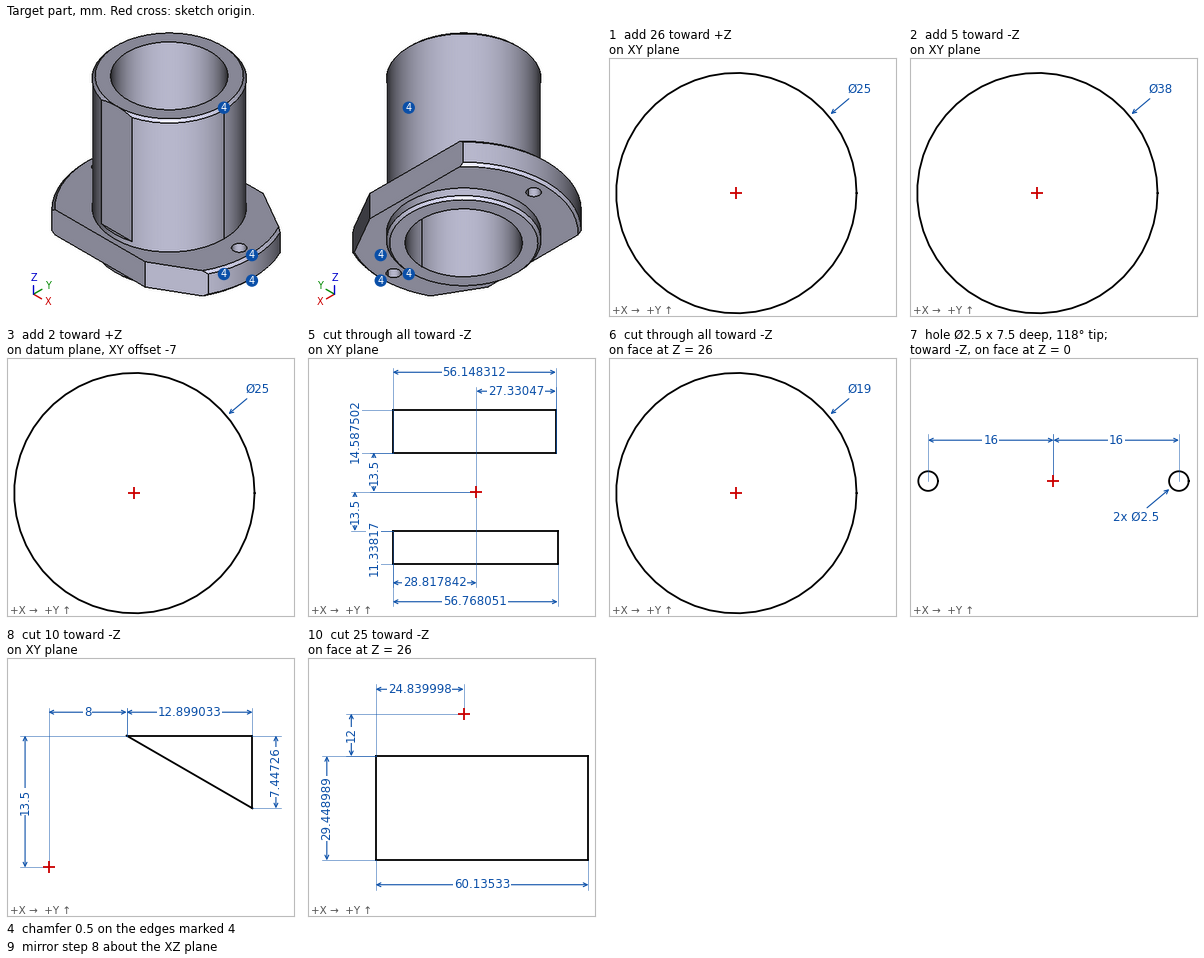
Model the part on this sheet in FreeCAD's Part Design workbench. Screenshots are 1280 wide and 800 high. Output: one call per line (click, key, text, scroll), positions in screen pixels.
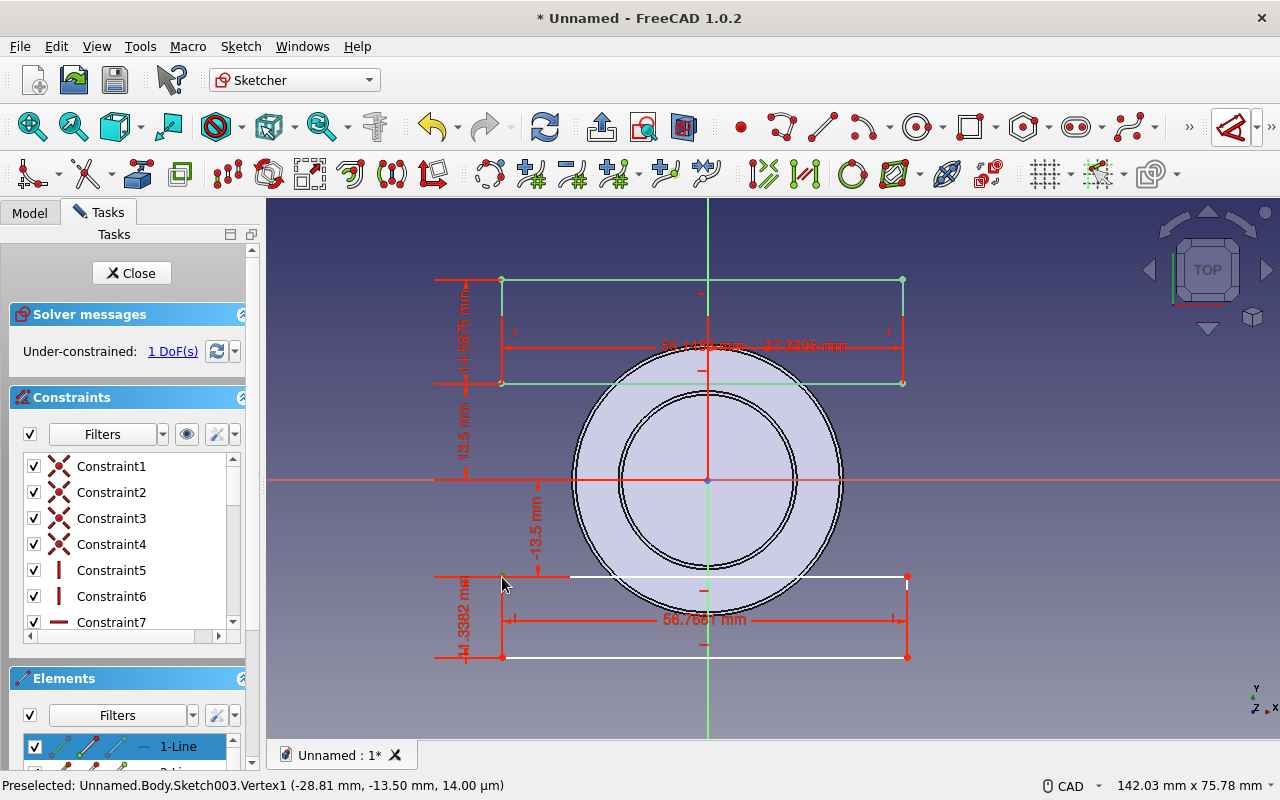
key(l)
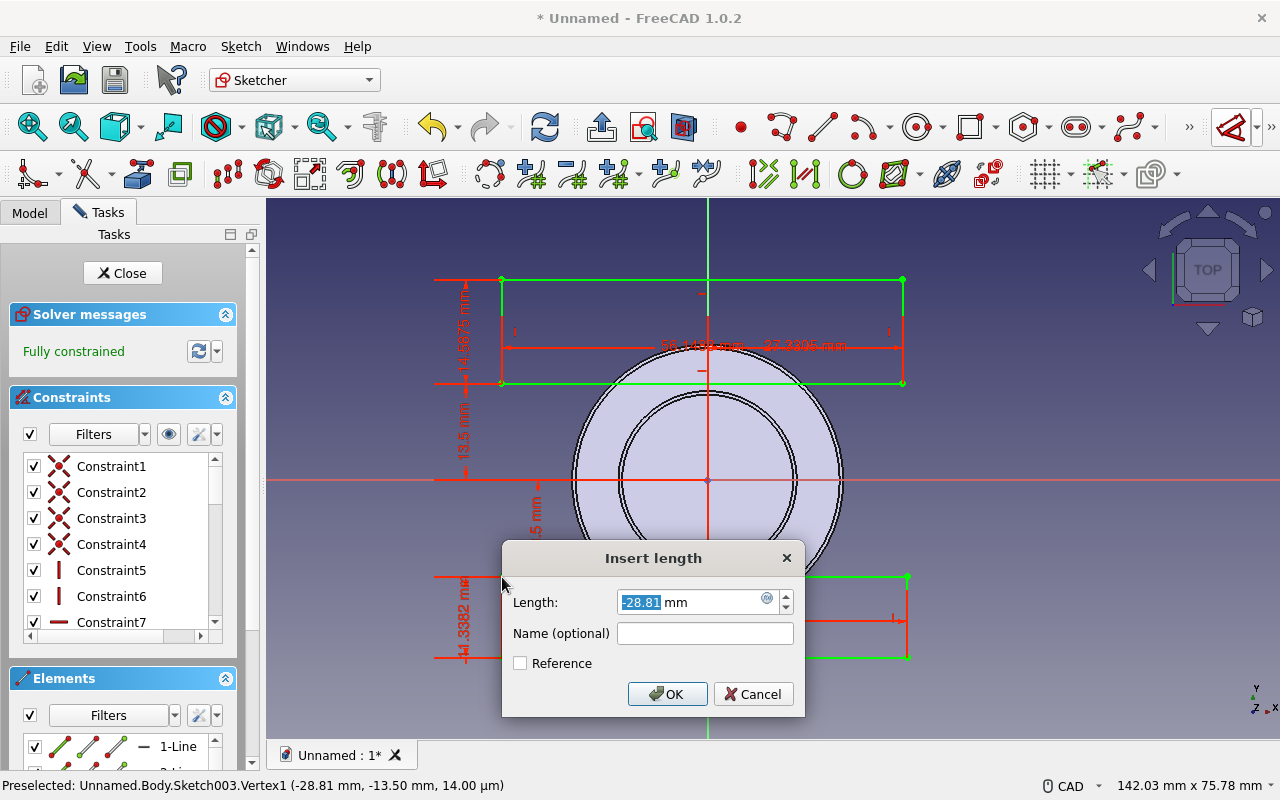
text(-28.817842)
key(Return)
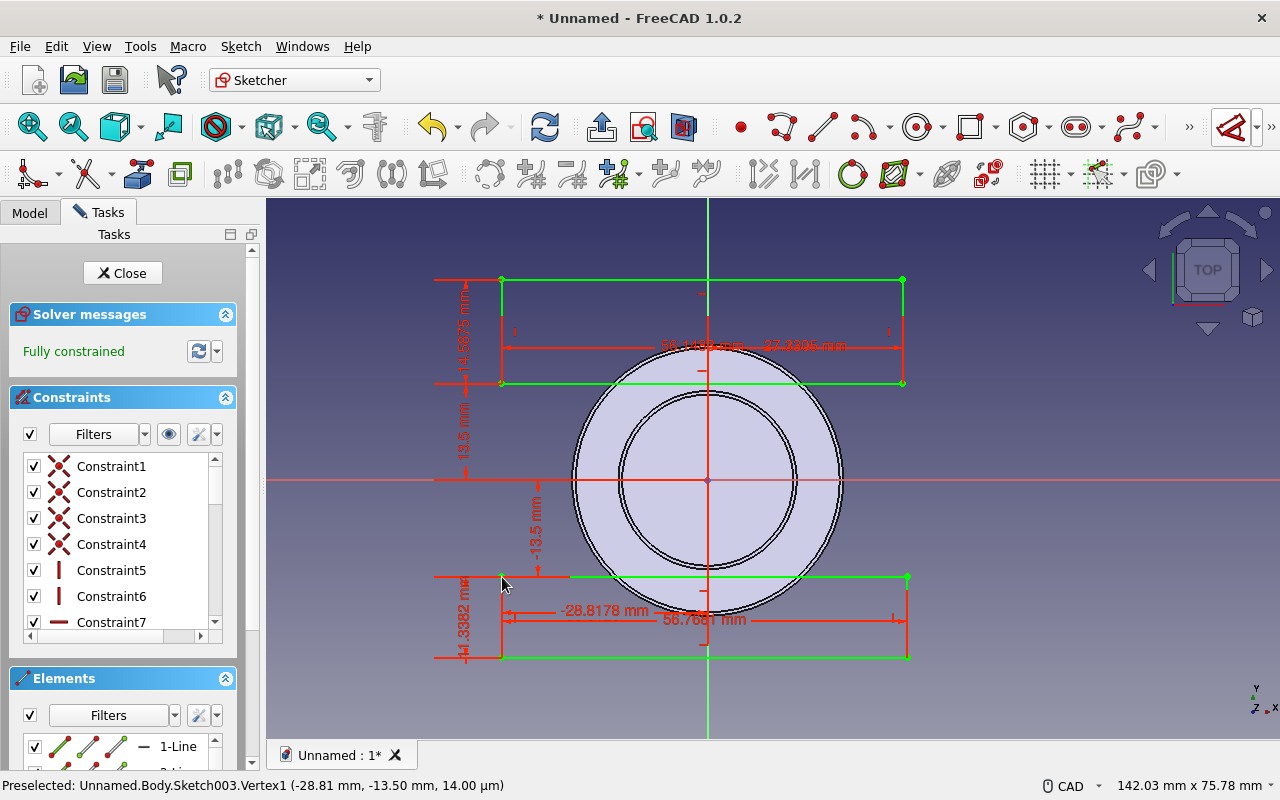
click(123, 273)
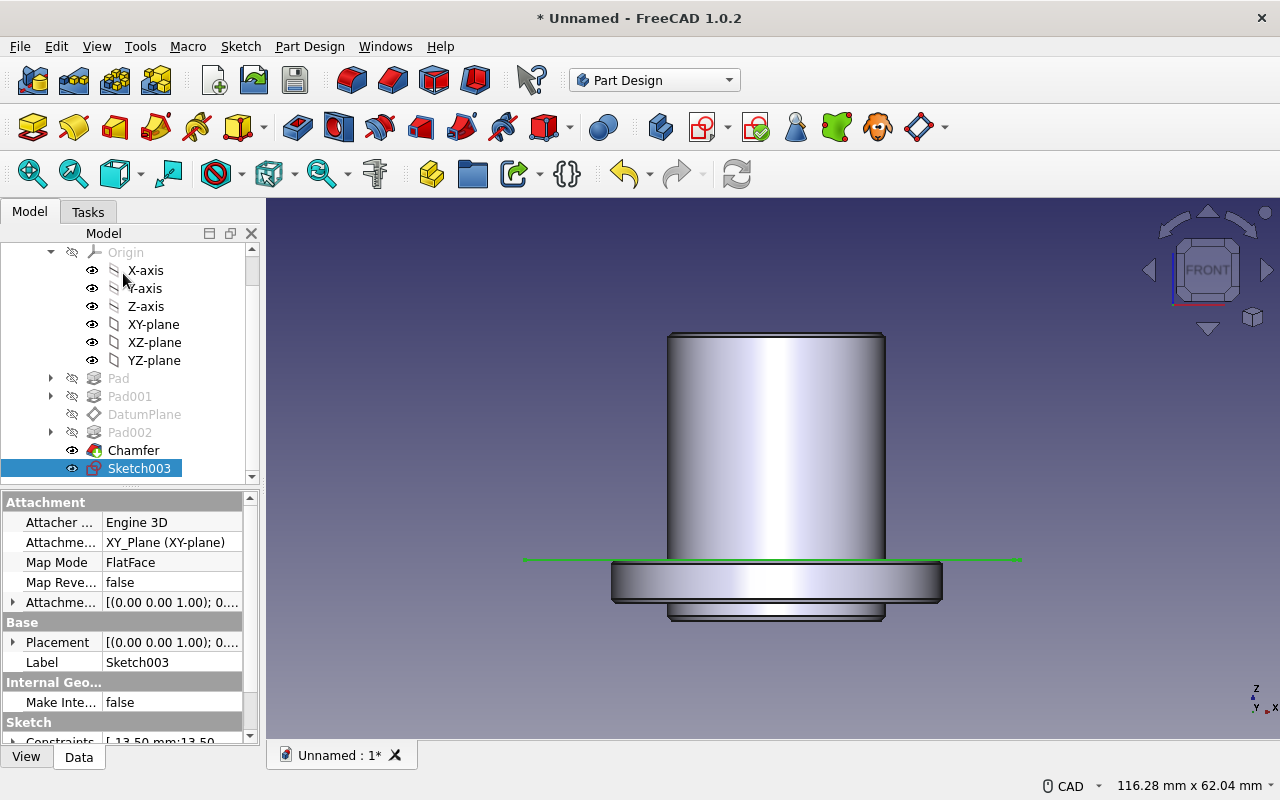
click(298, 128)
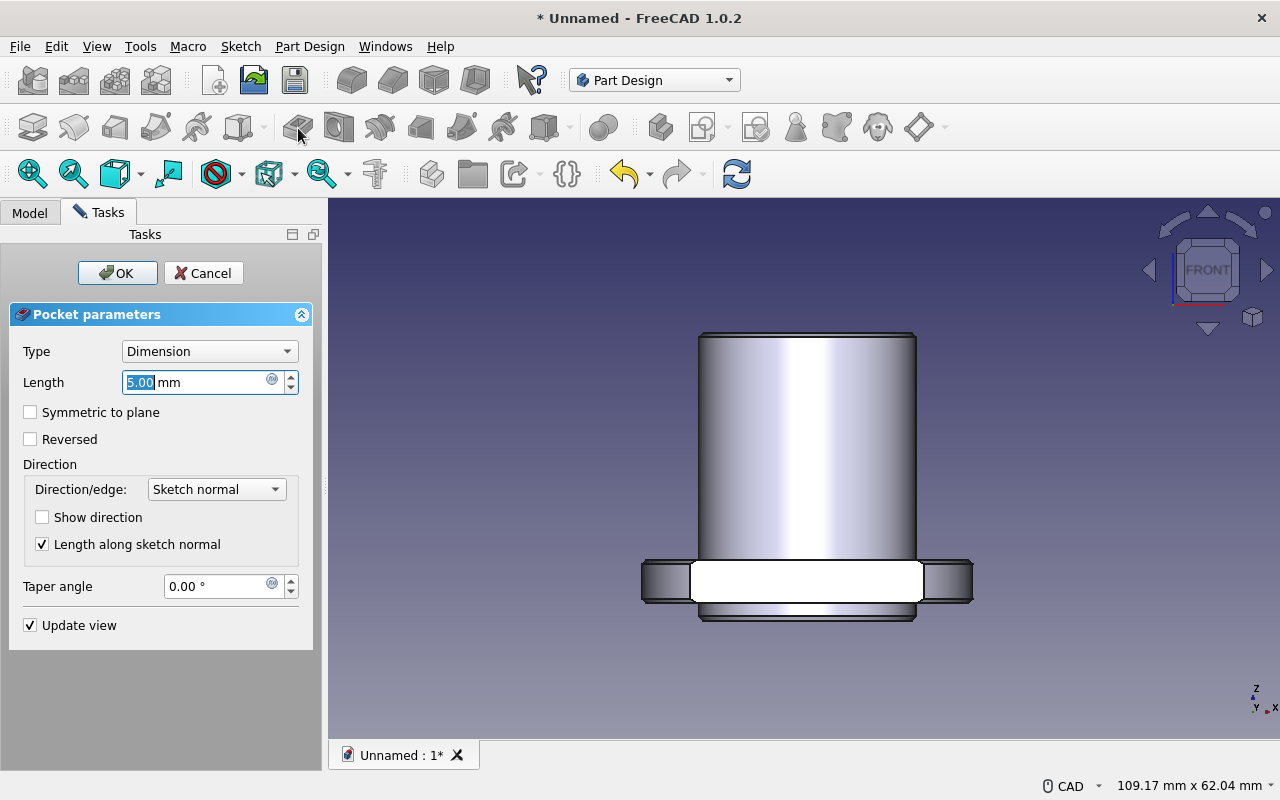
click(210, 352)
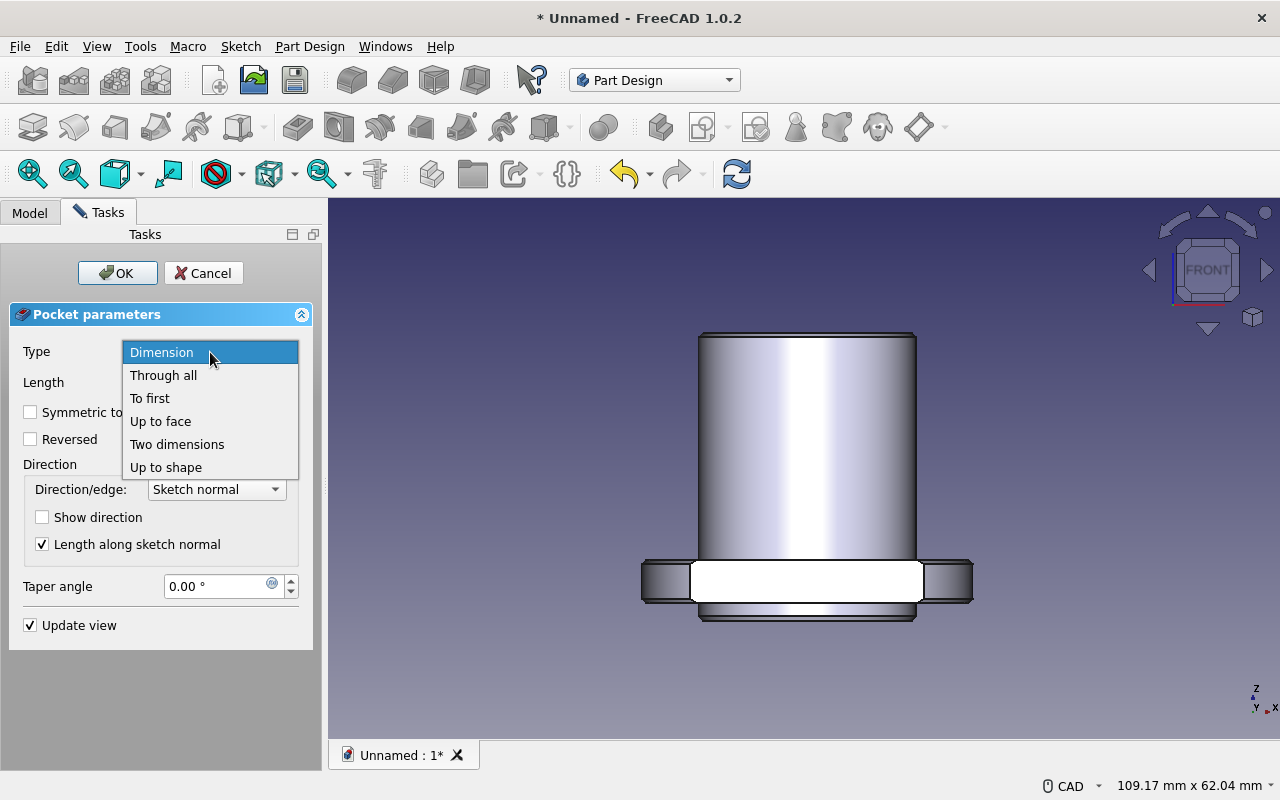
click(208, 376)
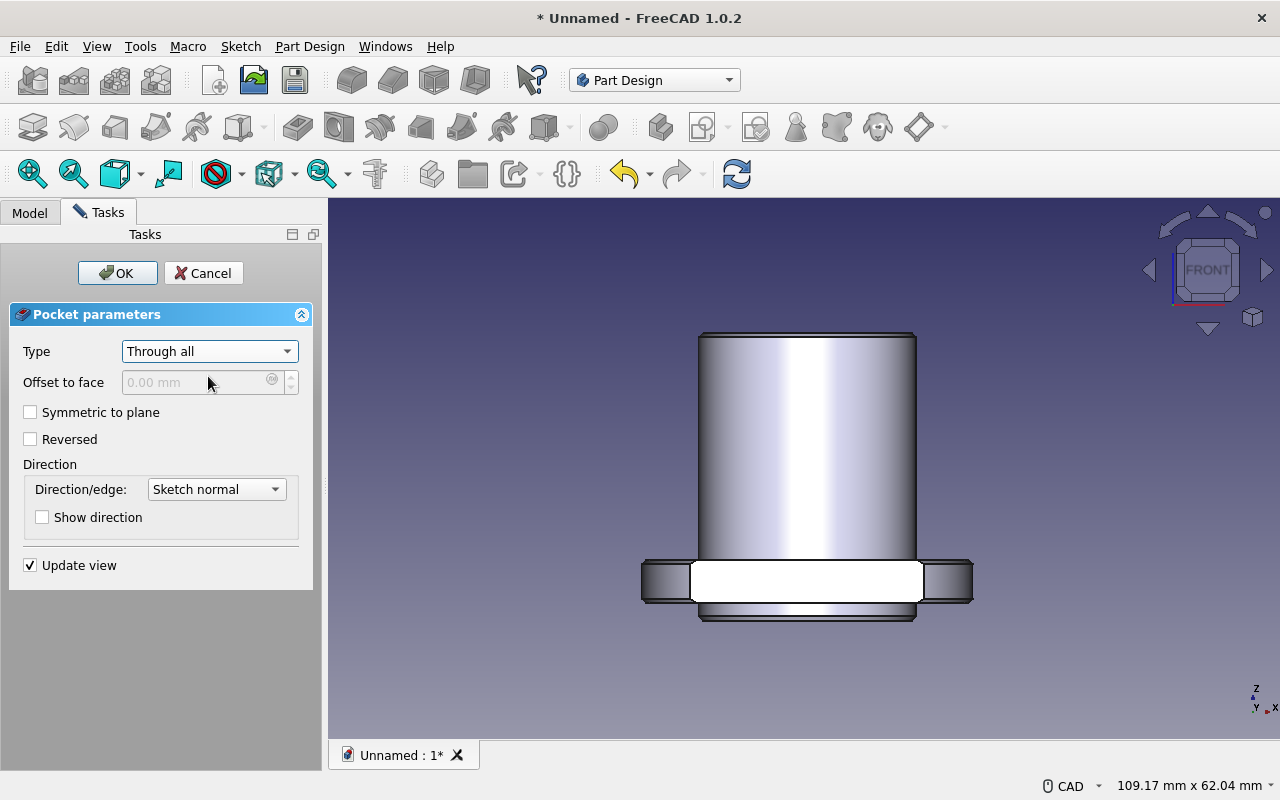
click(118, 273)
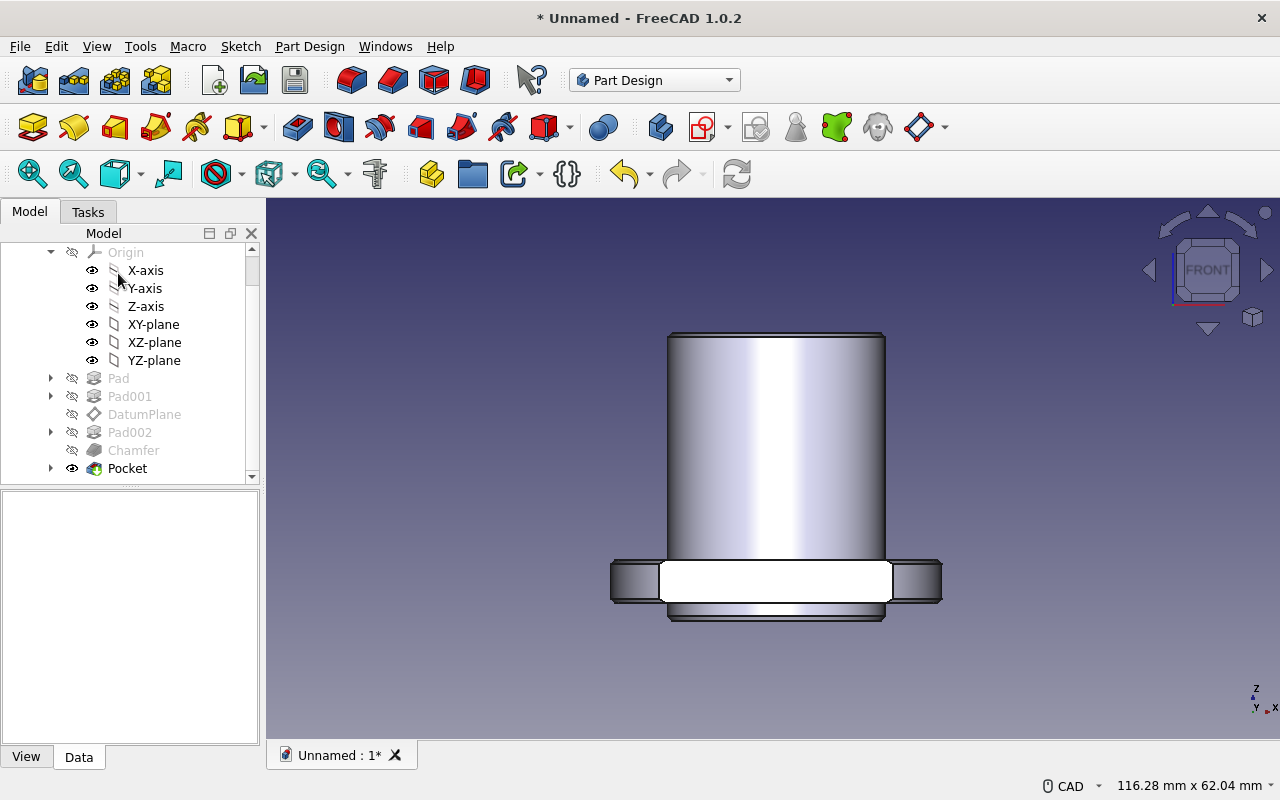
key(0)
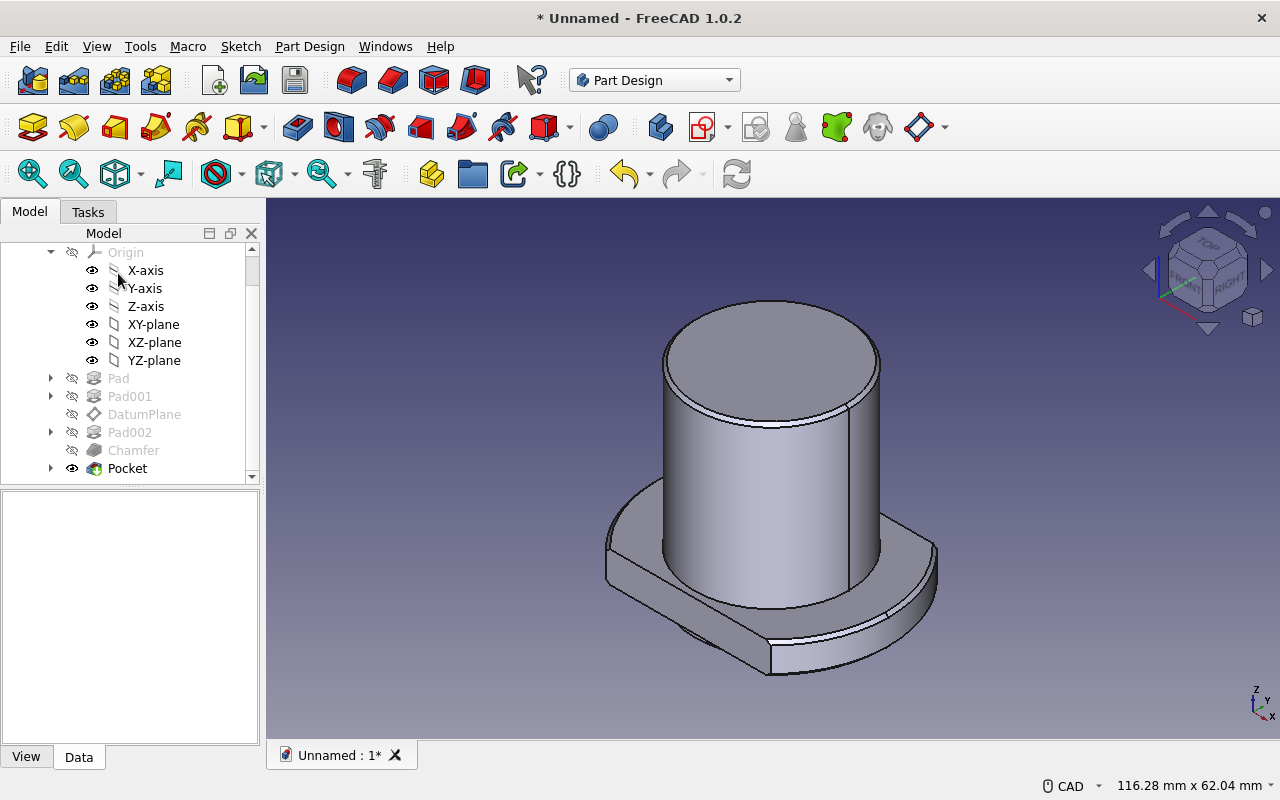
click(771, 360)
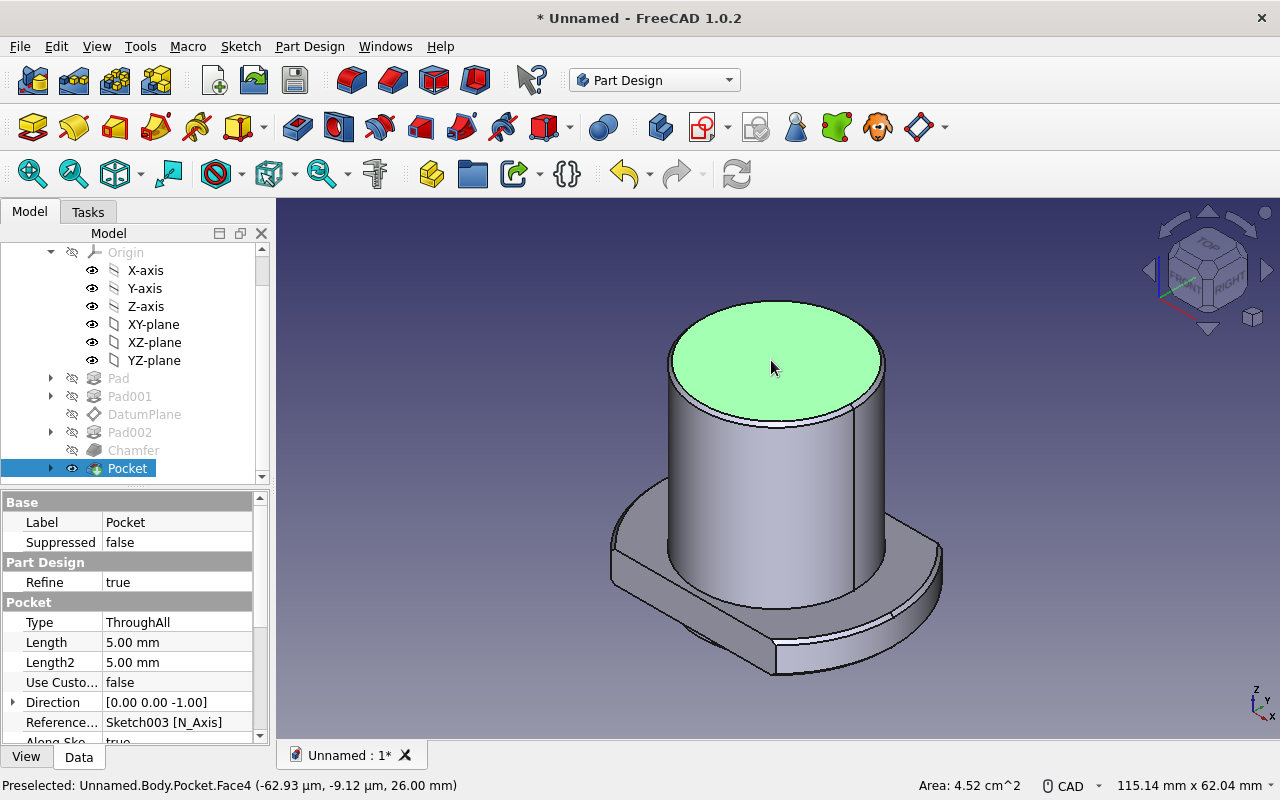
click(702, 128)